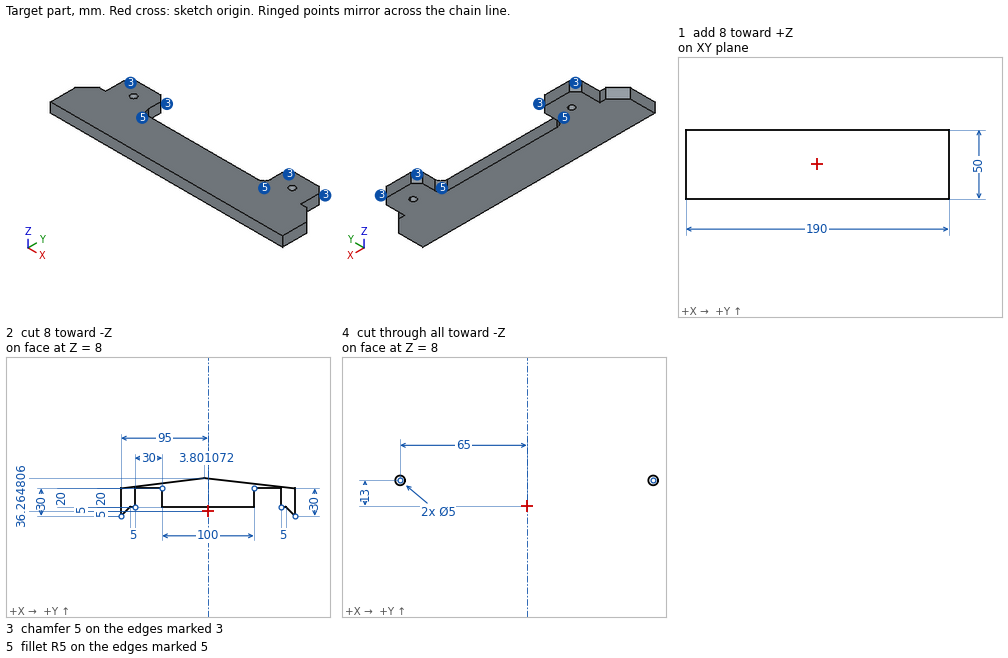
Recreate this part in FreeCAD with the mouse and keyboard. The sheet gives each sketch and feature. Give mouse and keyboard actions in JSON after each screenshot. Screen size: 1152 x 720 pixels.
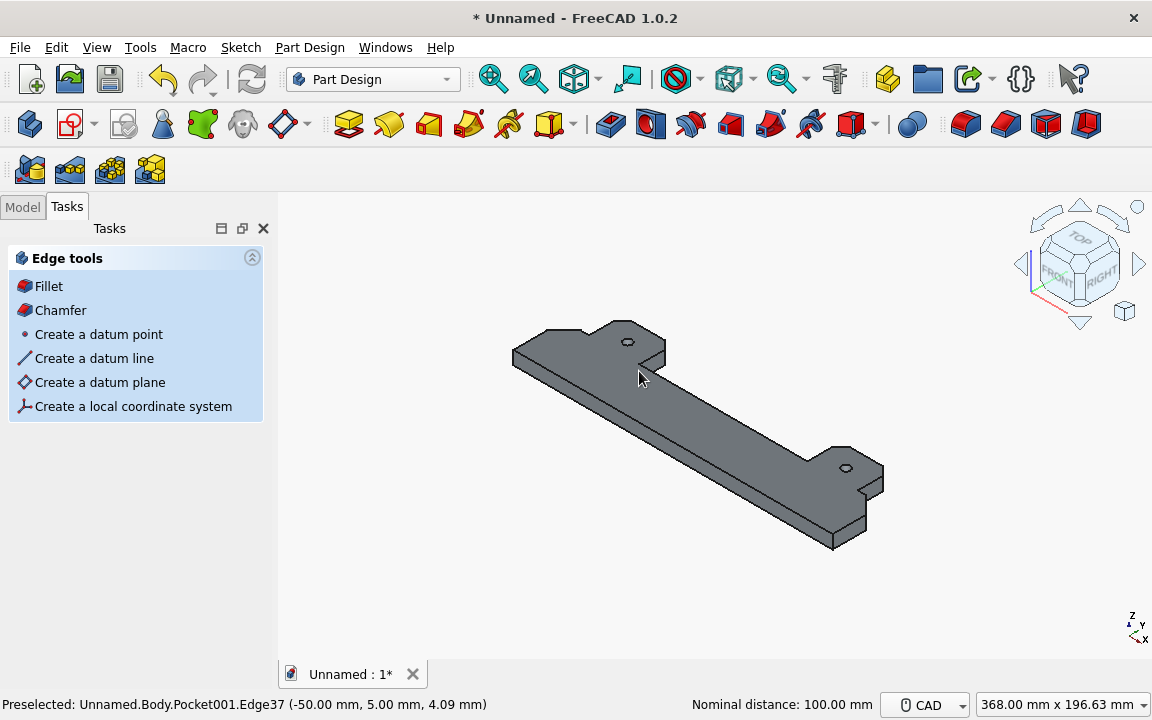
{"action": "left_click", "coordinate": [966, 124]}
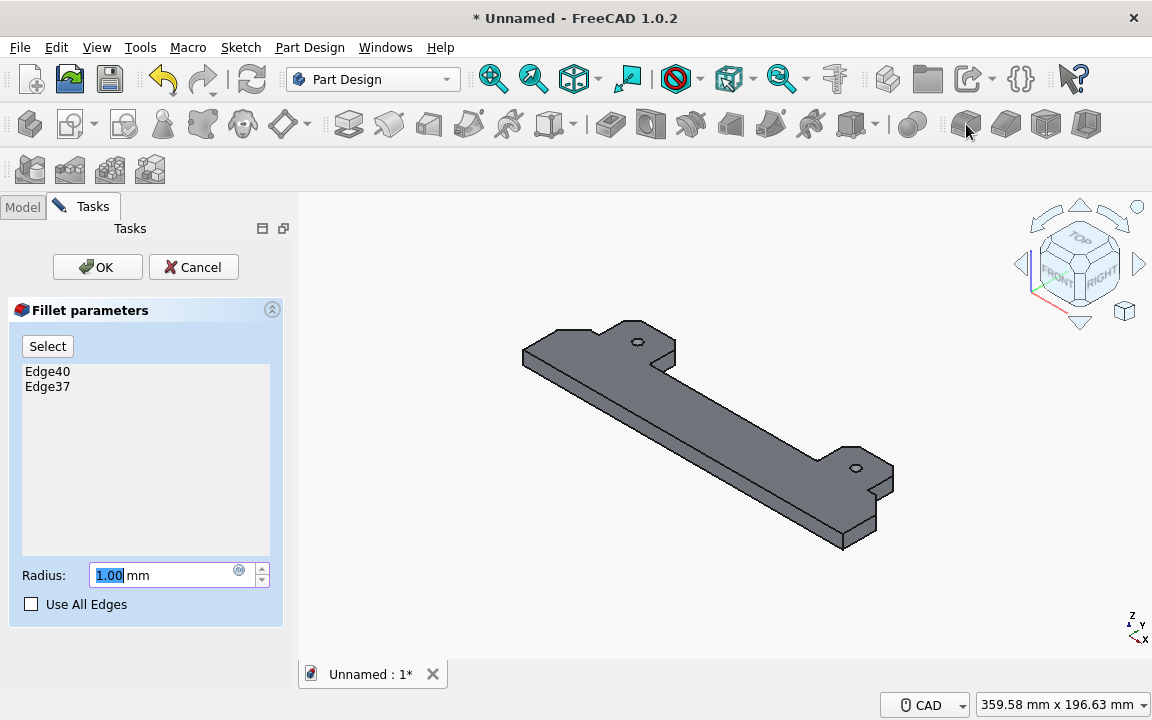
{"action": "type", "text": "5"}
{"action": "key", "text": "Tab"}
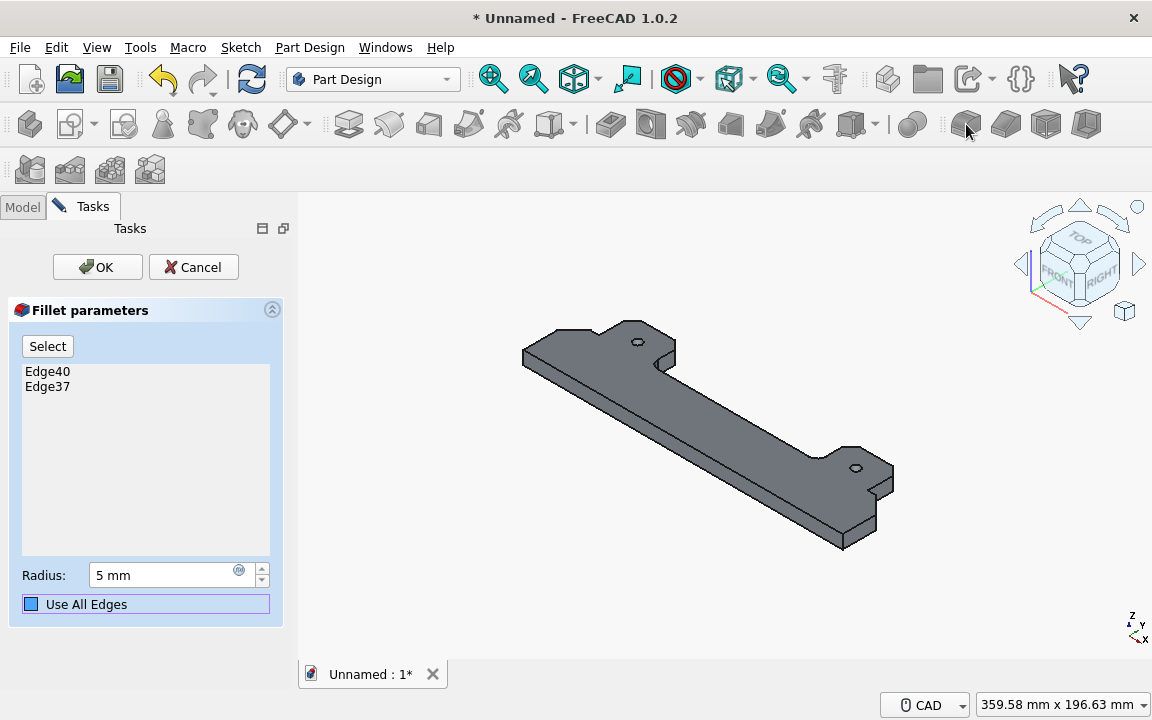
{"action": "left_click", "coordinate": [98, 267]}